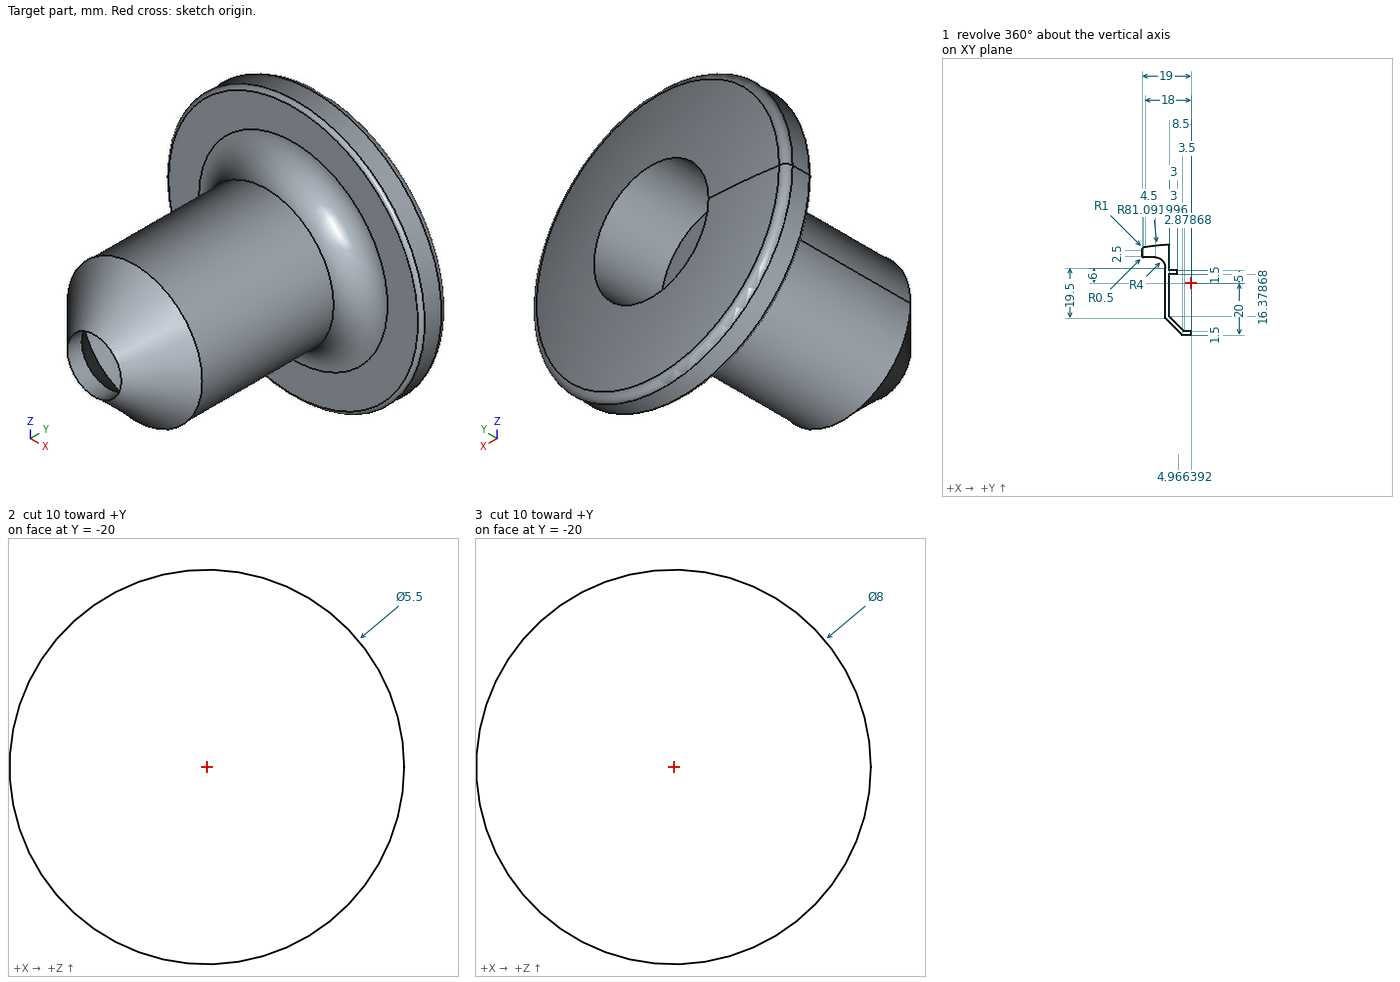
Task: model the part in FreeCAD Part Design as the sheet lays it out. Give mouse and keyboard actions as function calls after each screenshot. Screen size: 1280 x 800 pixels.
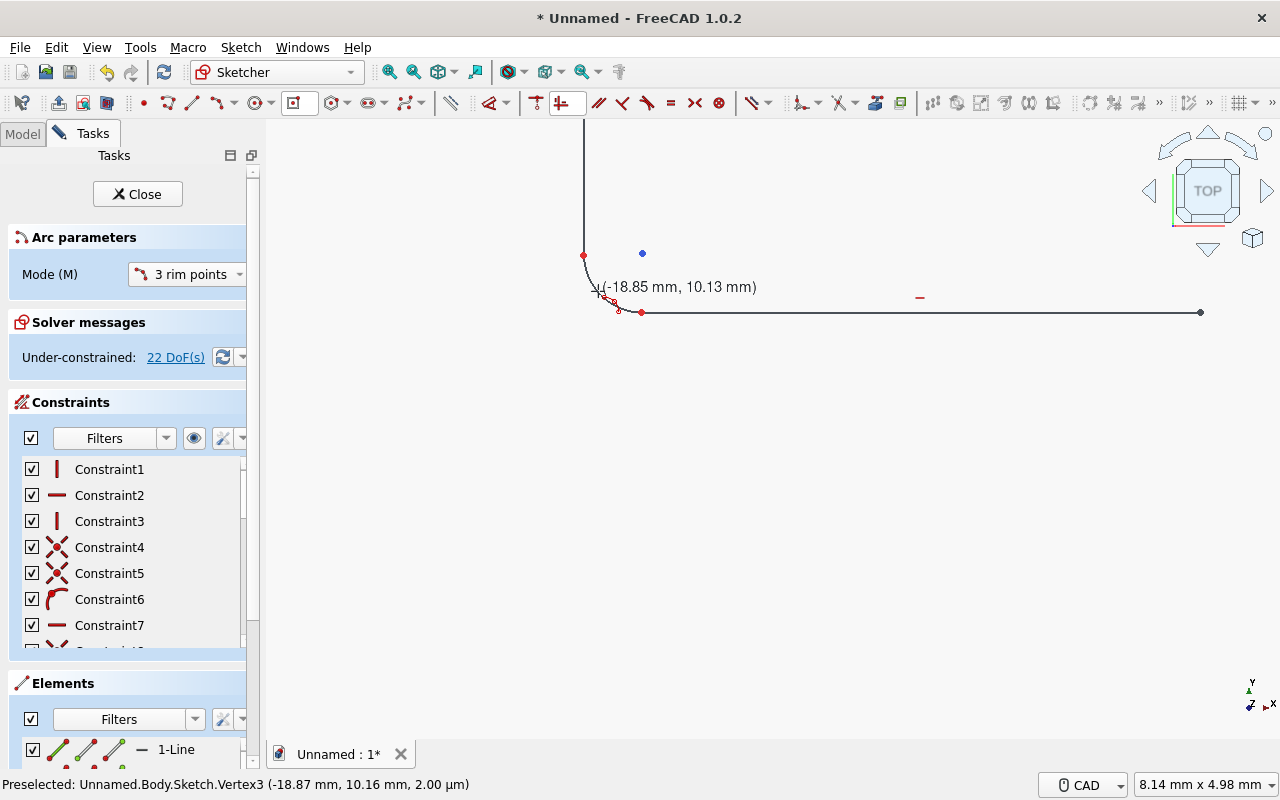
scroll(599, 286, down, 12)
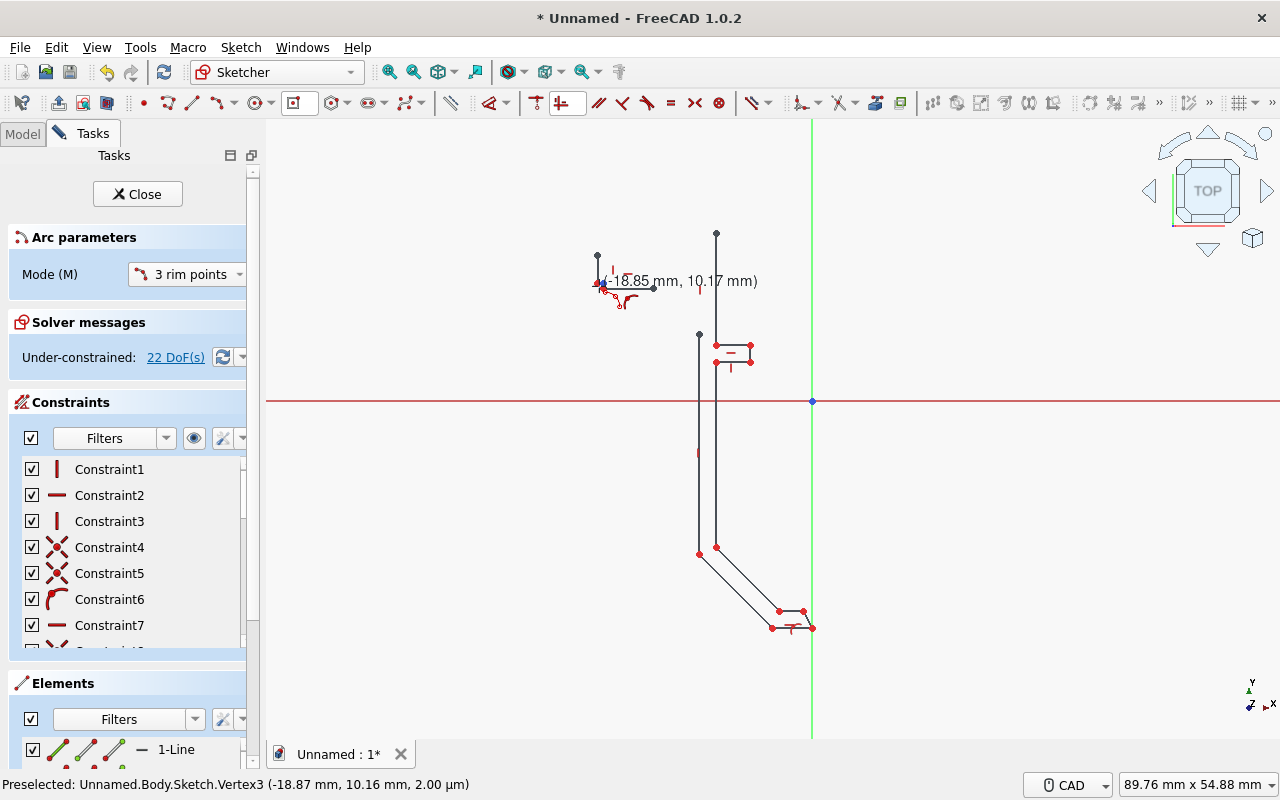
click(654, 289)
click(699, 334)
click(686, 302)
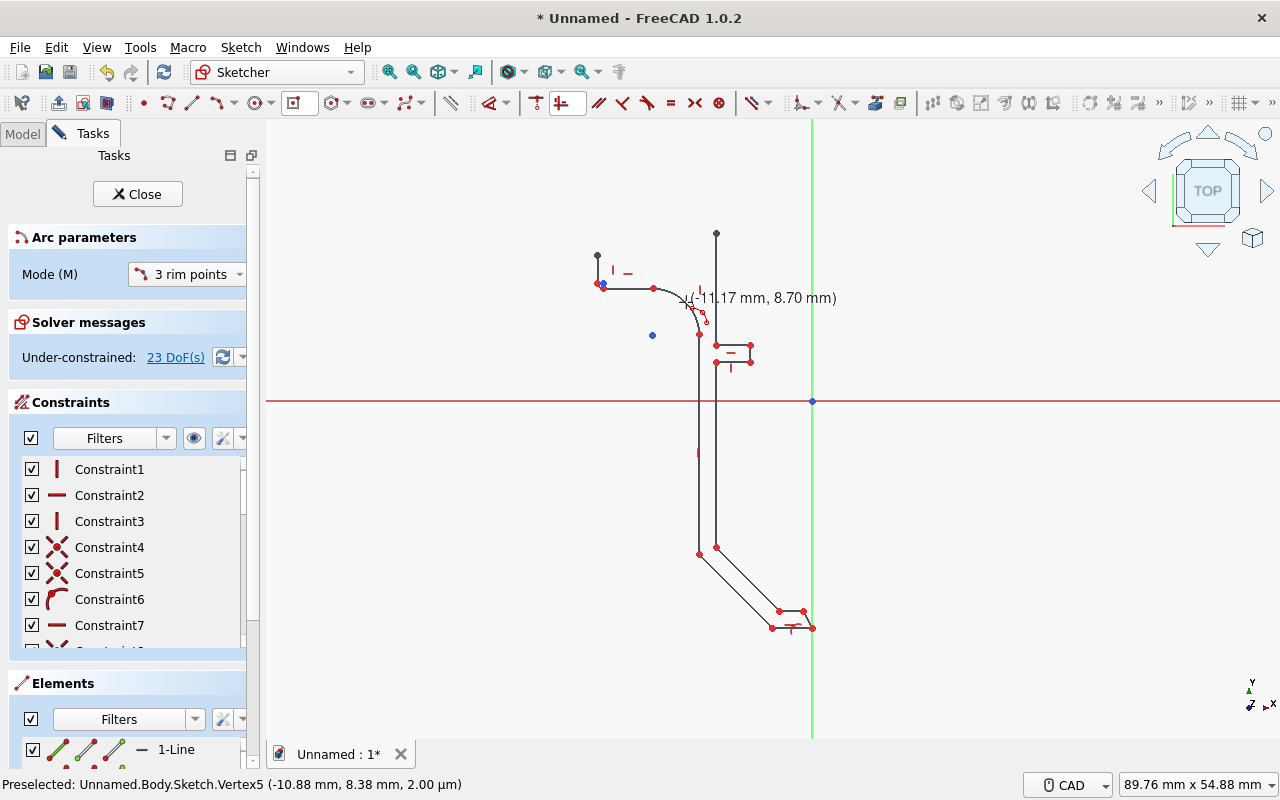
click(716, 233)
click(609, 243)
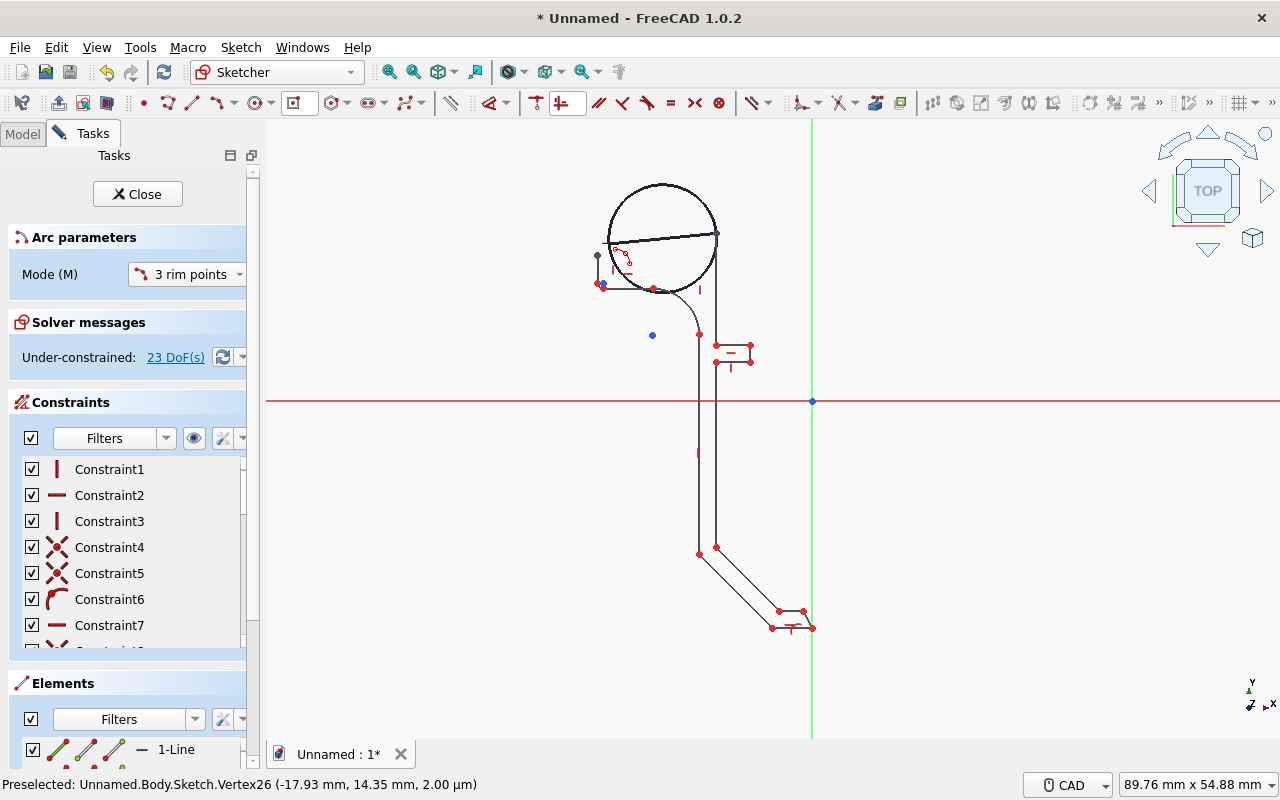
scroll(662, 236, up, 12)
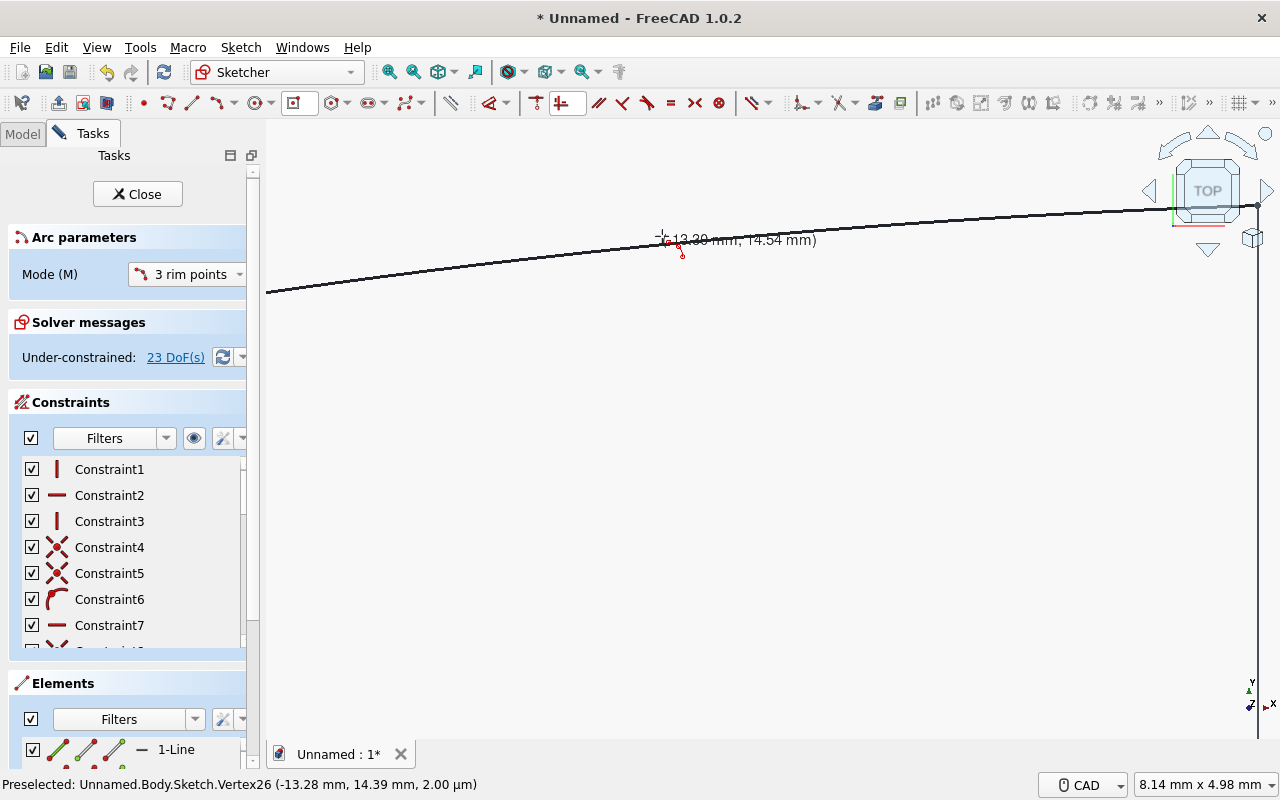
click(662, 234)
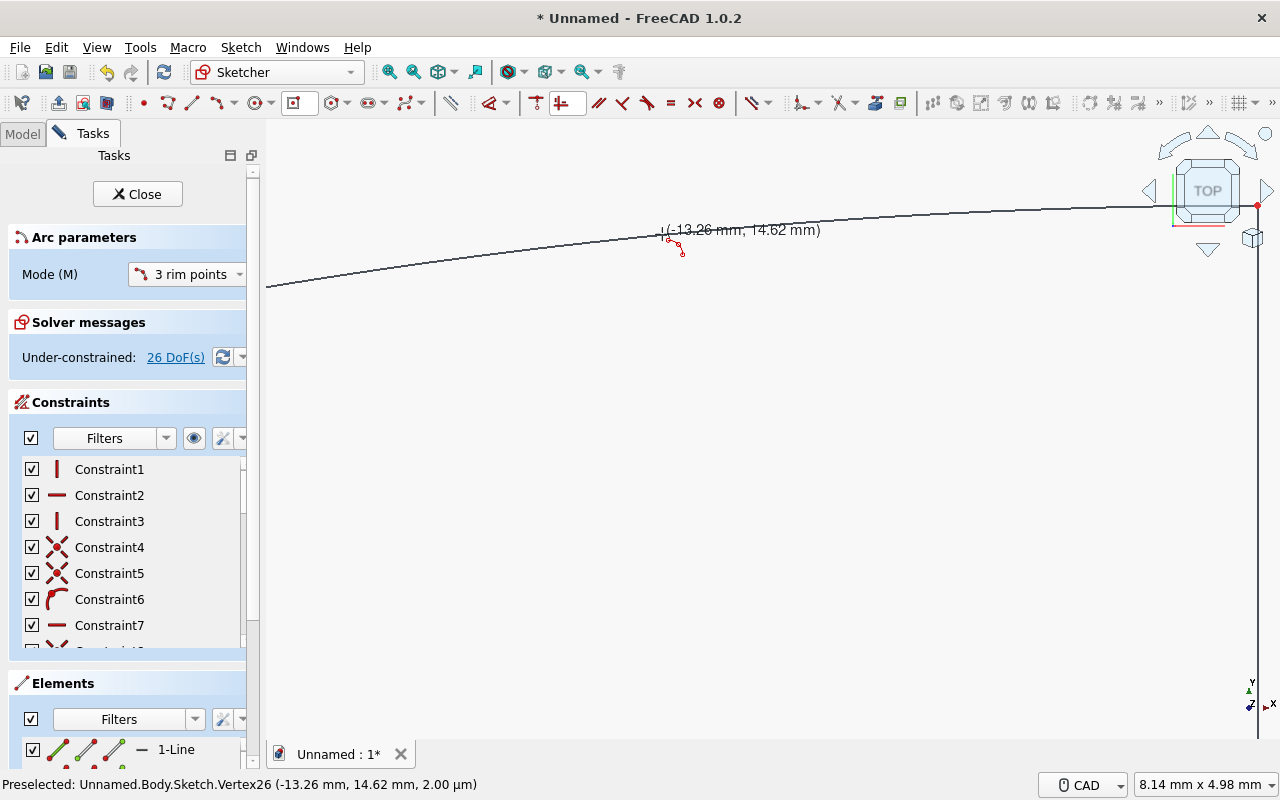
scroll(662, 235, down, 12)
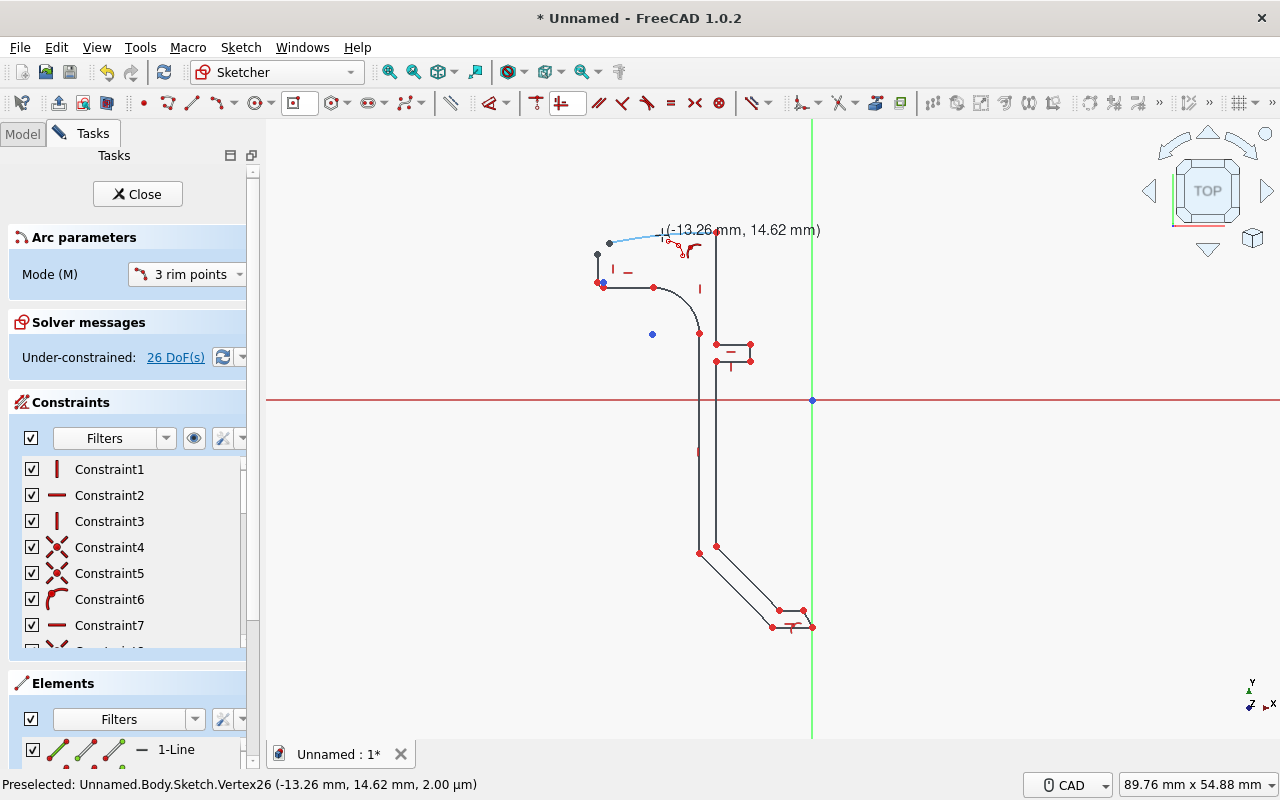
click(609, 243)
click(598, 255)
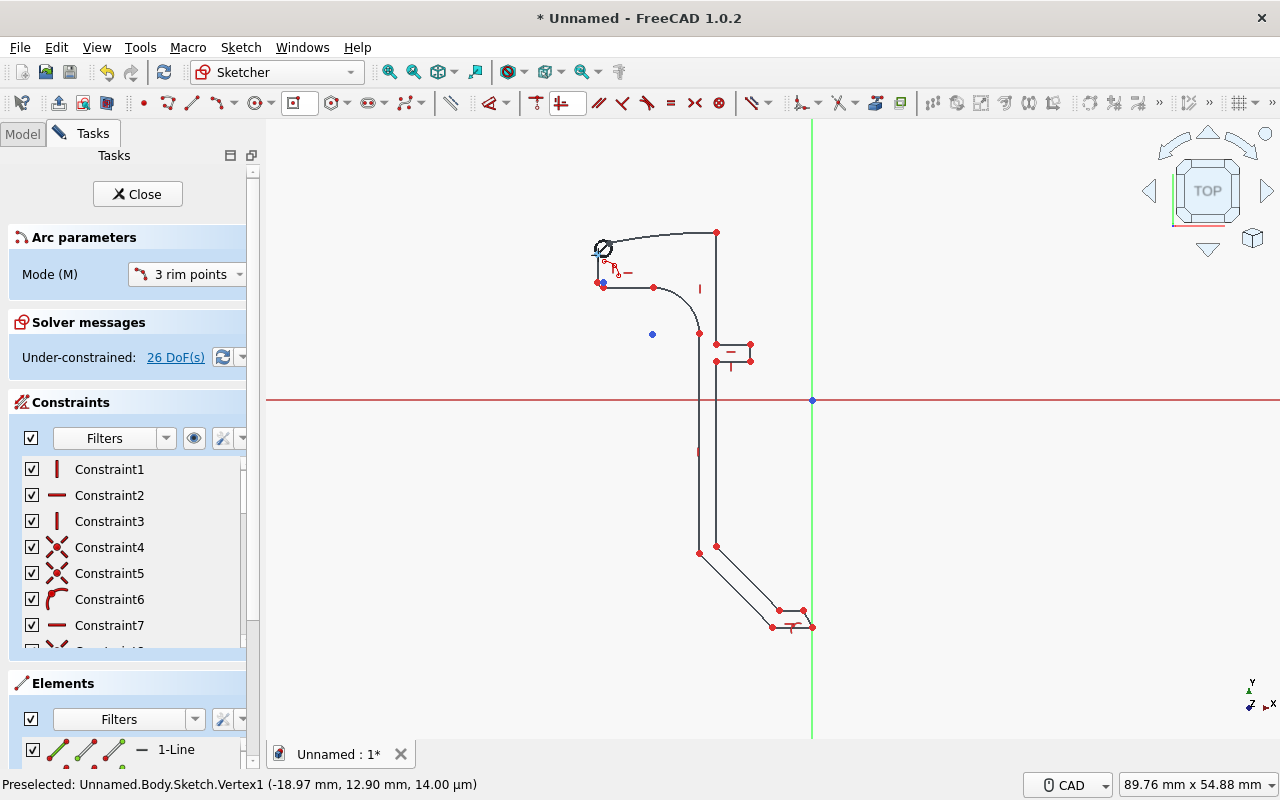
scroll(601, 246, up, 8)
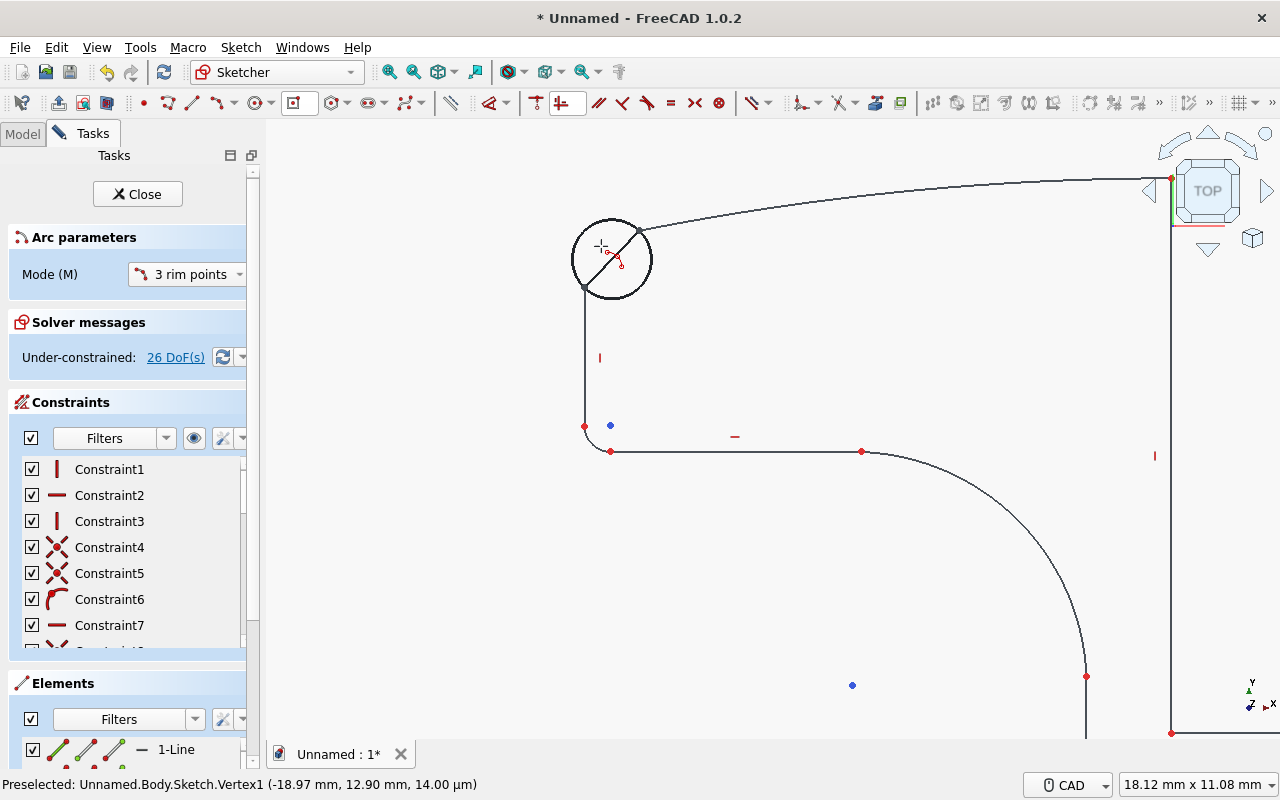
click(599, 243)
key(Escape)